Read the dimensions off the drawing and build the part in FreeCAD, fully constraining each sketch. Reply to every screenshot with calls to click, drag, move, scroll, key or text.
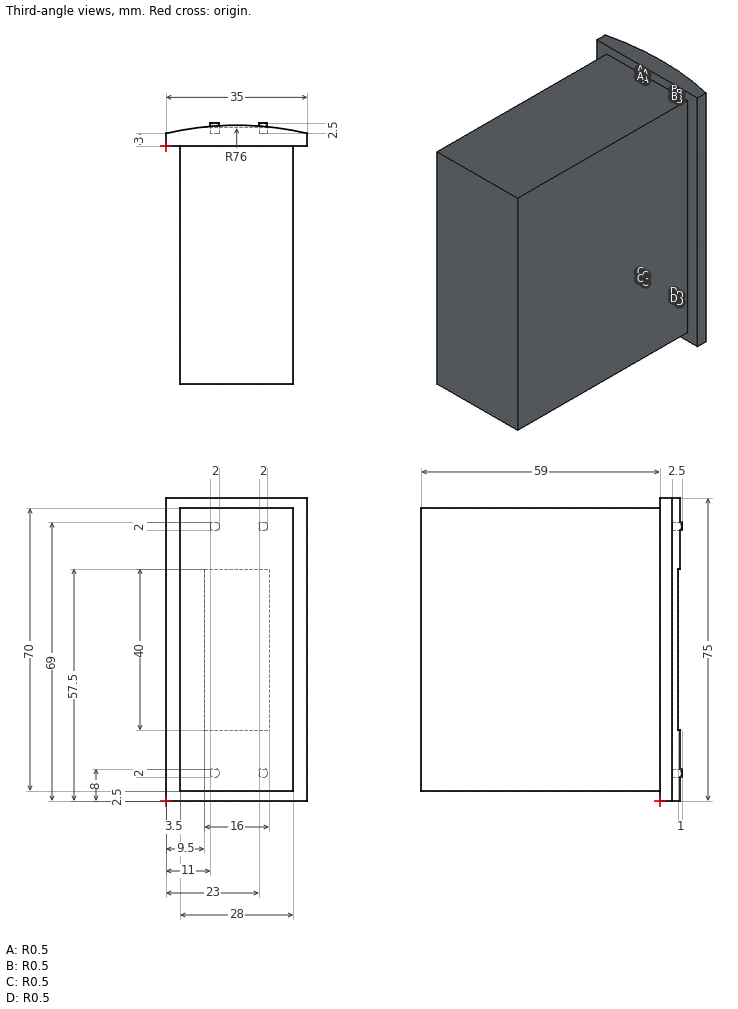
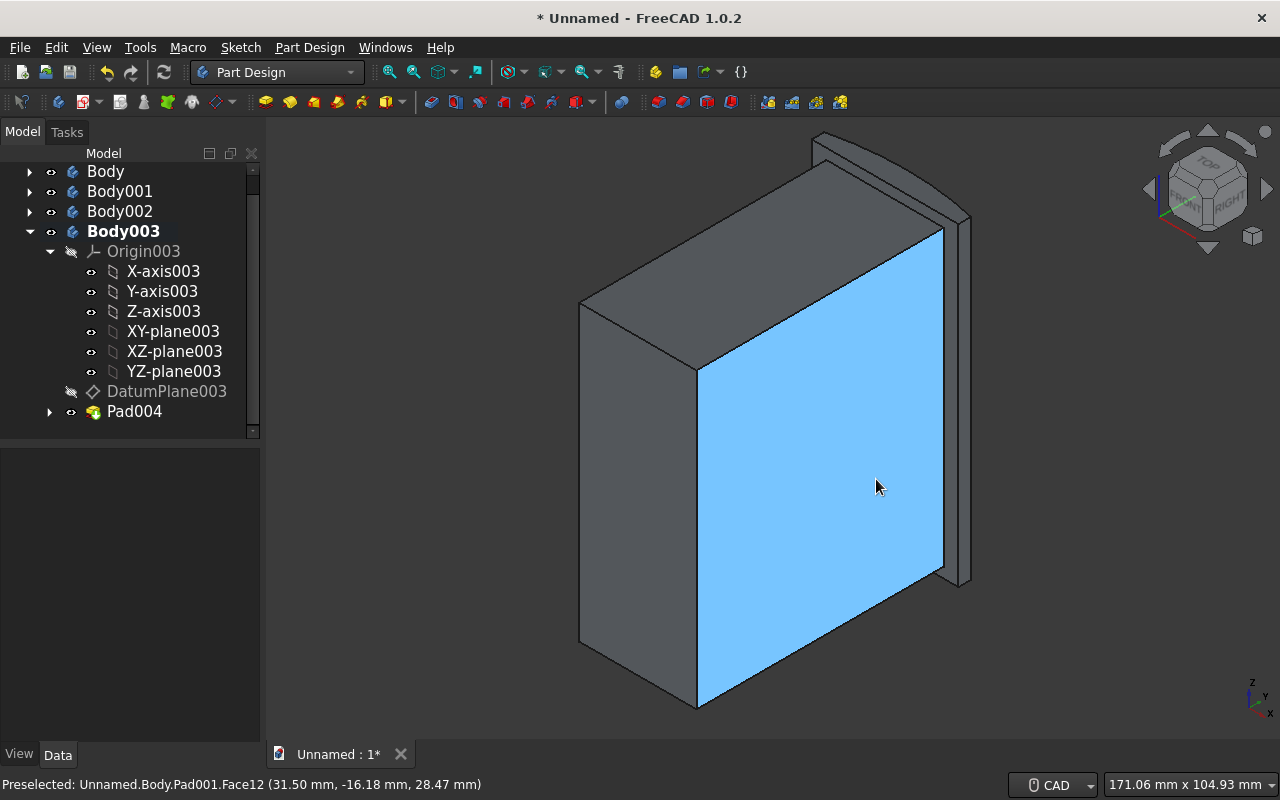
key(2)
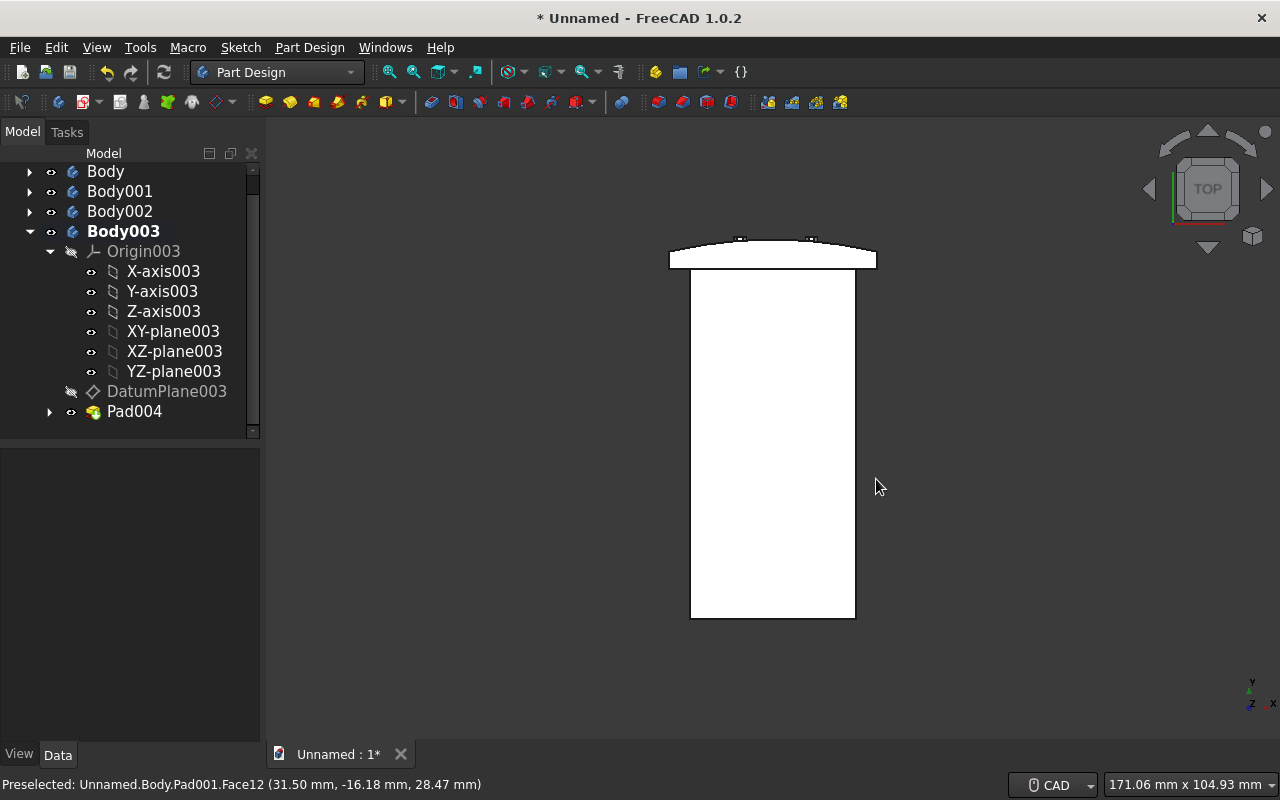
key(v)
key(f)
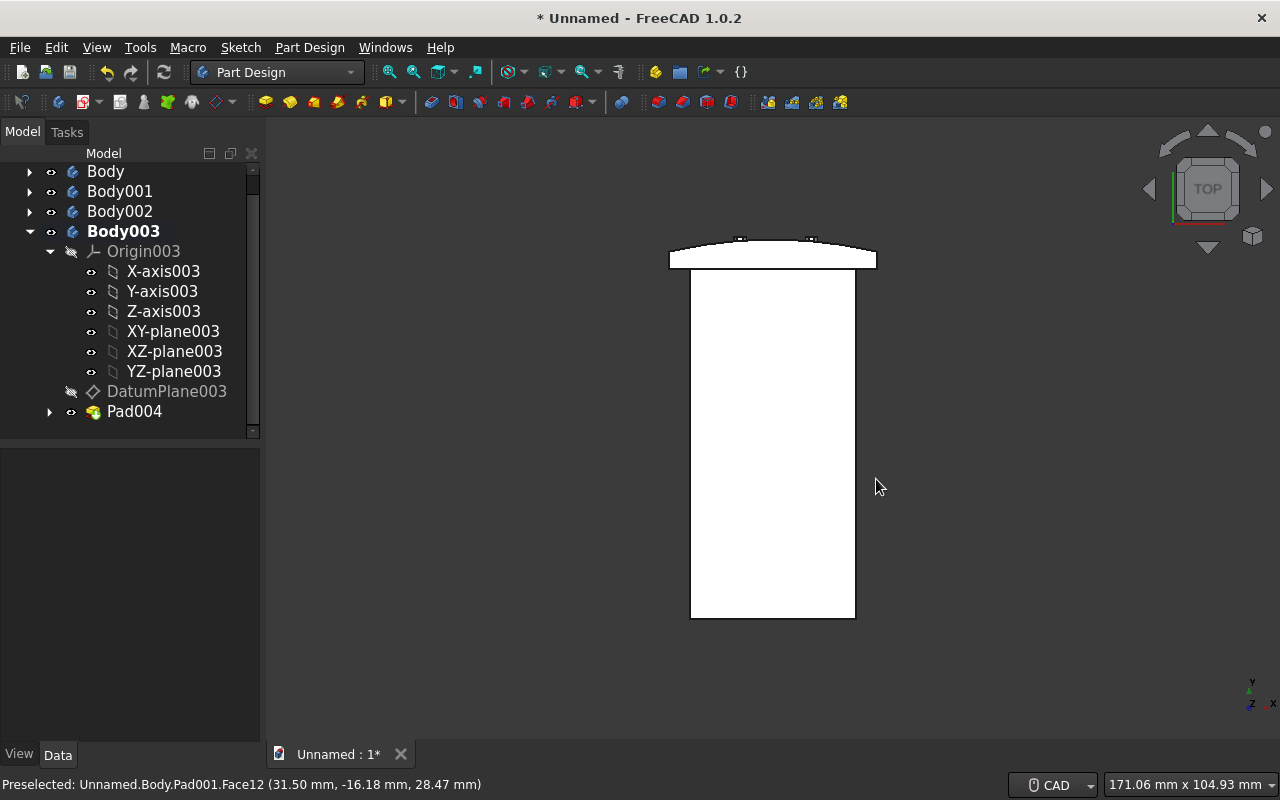
scroll(734, 243, up, 5)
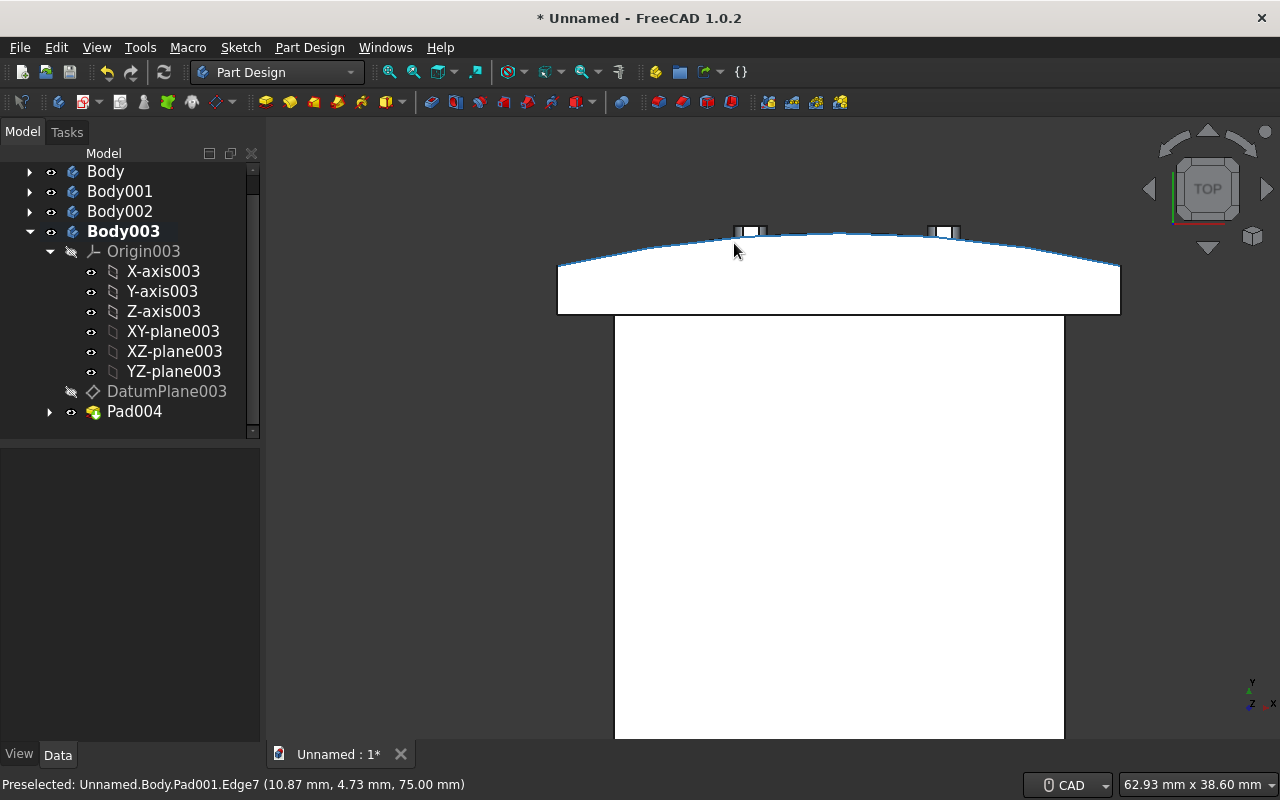
key(v)
key(f)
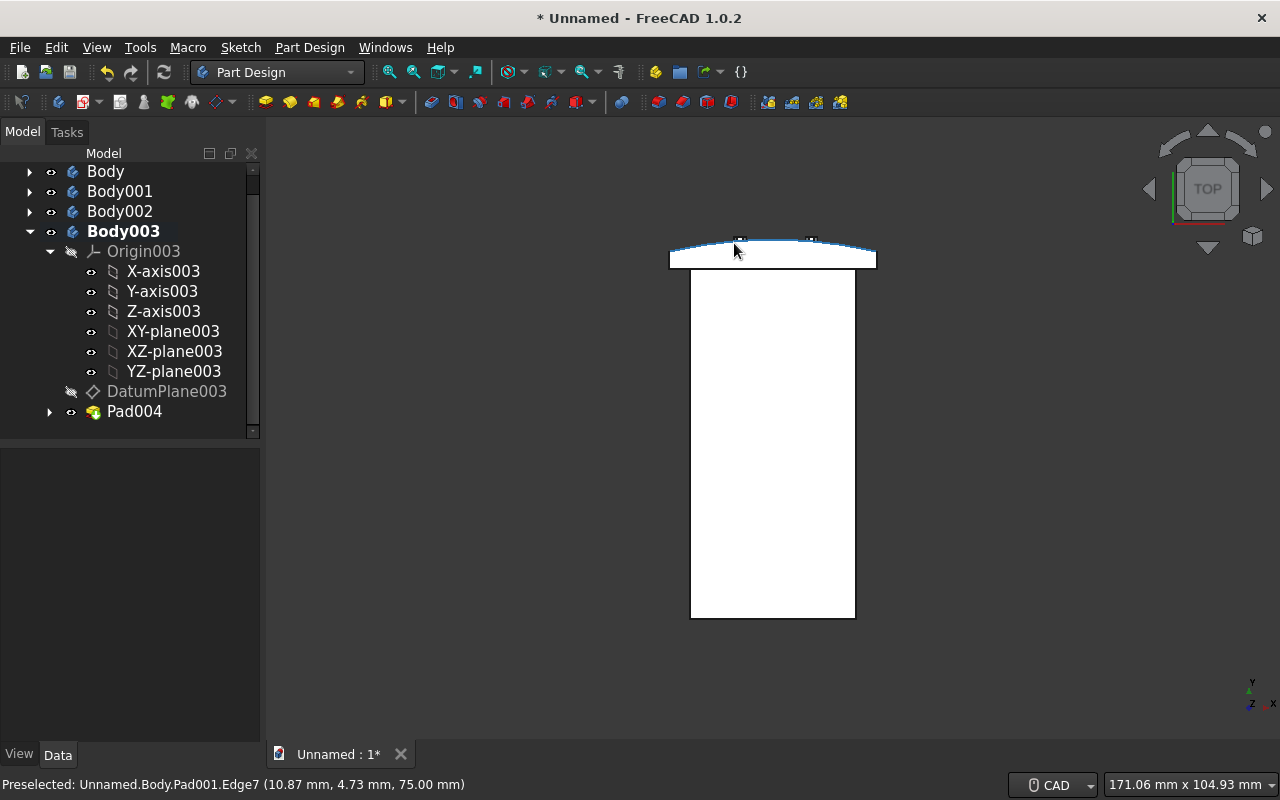
key(0)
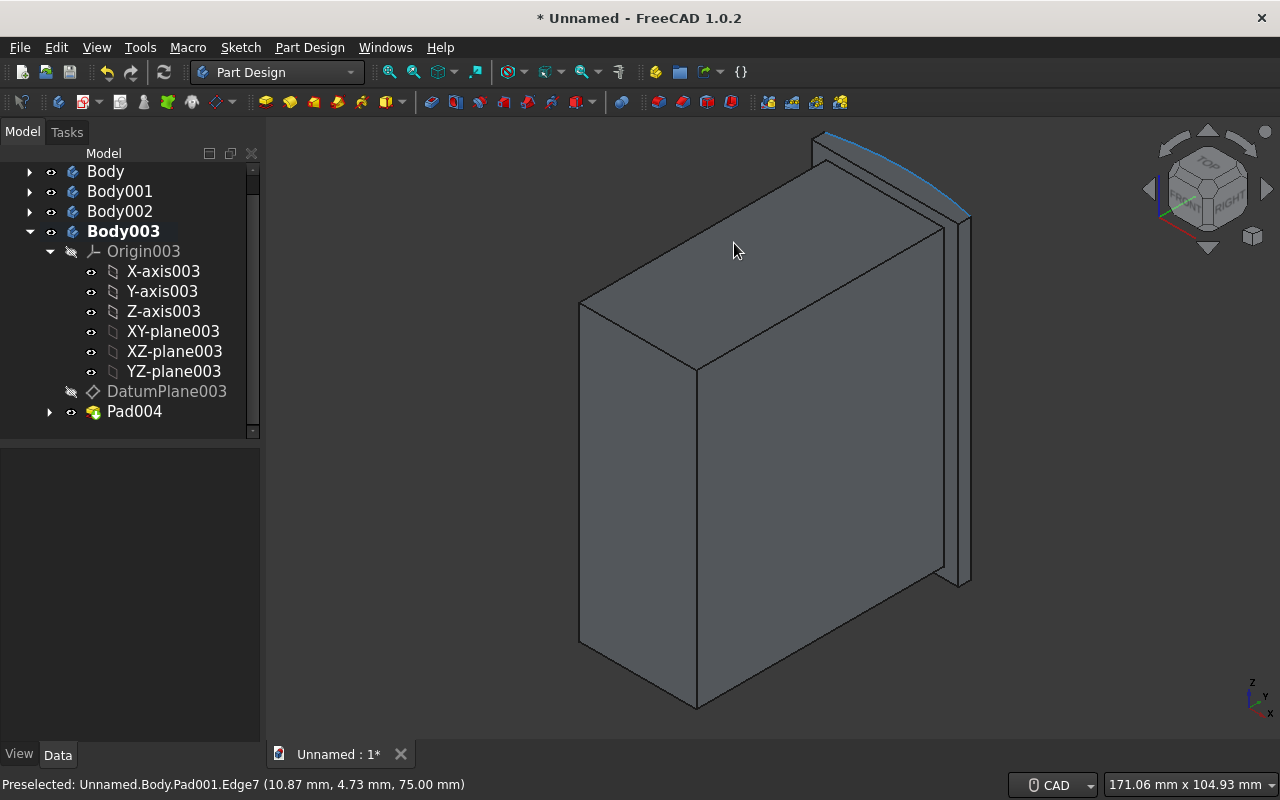
key(v)
key(f)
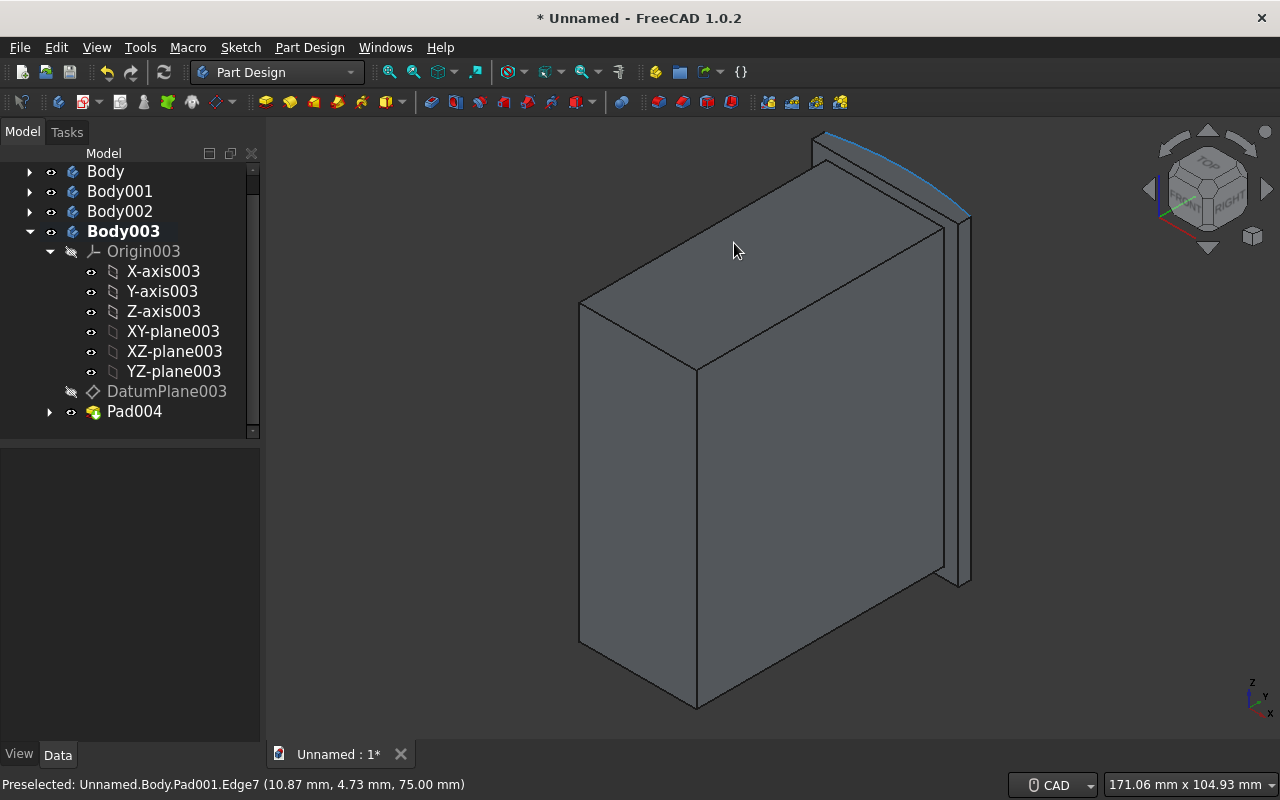
scroll(876, 479, up, 5)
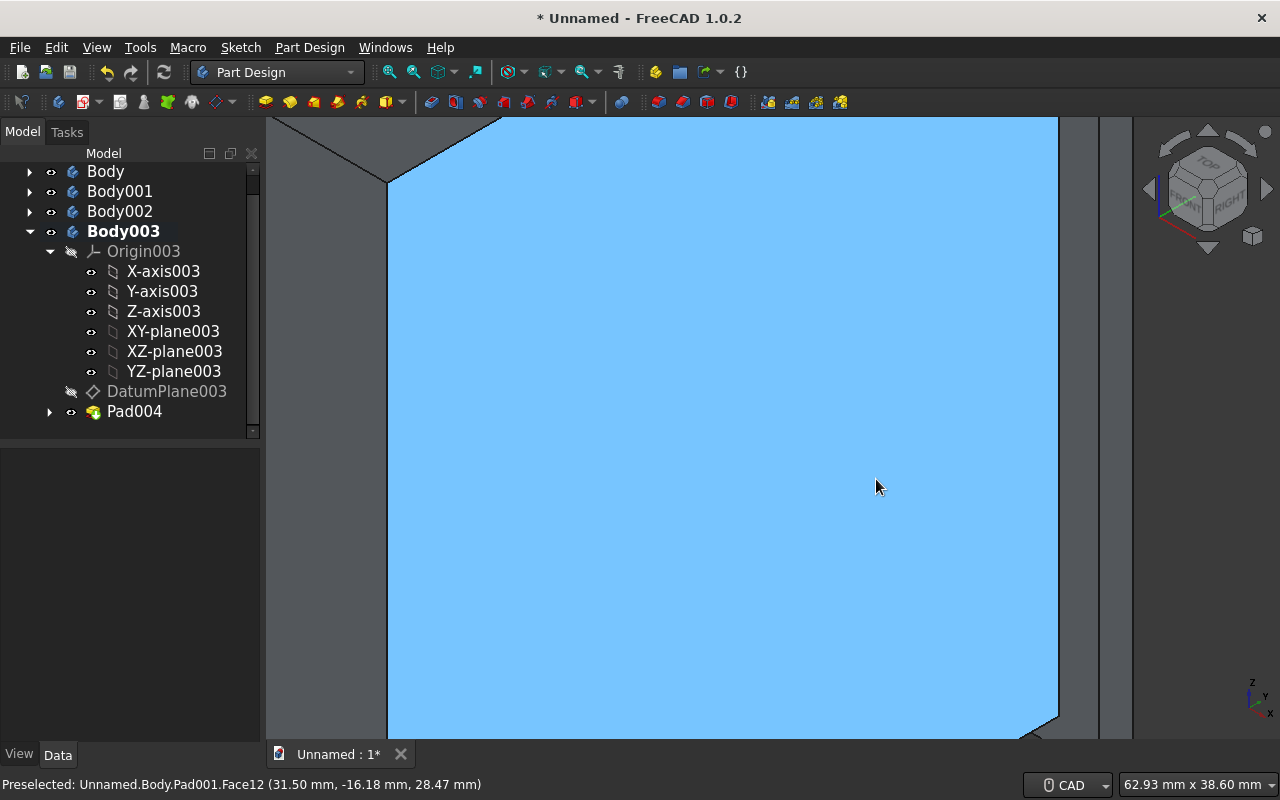
key(v)
key(f)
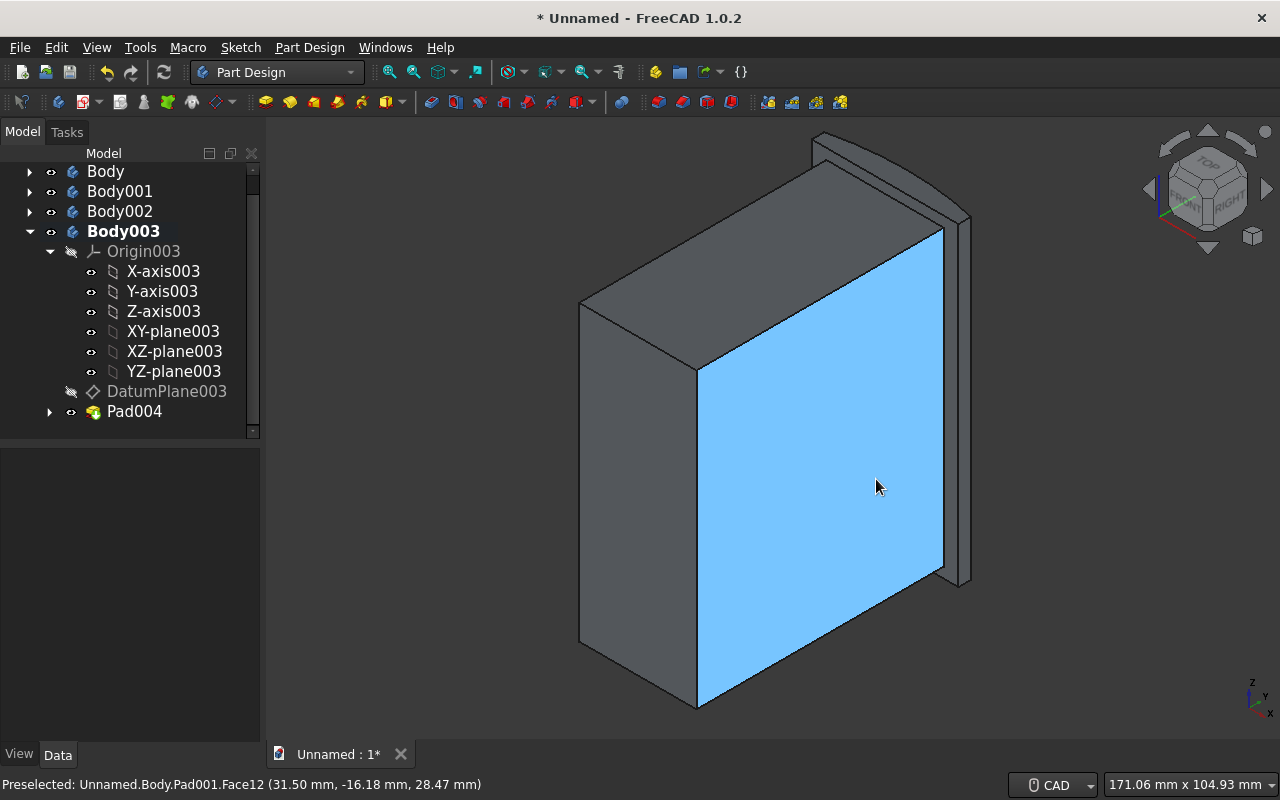
key(1)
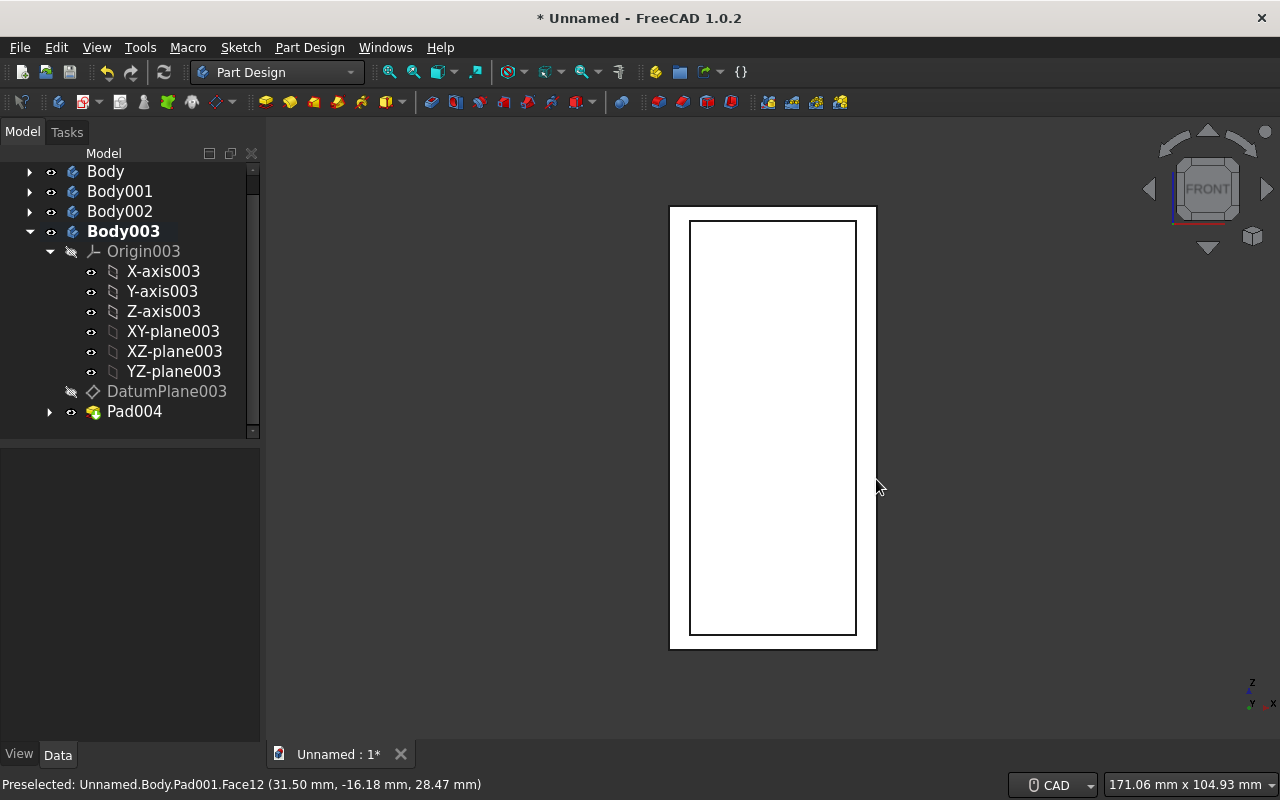
click(390, 72)